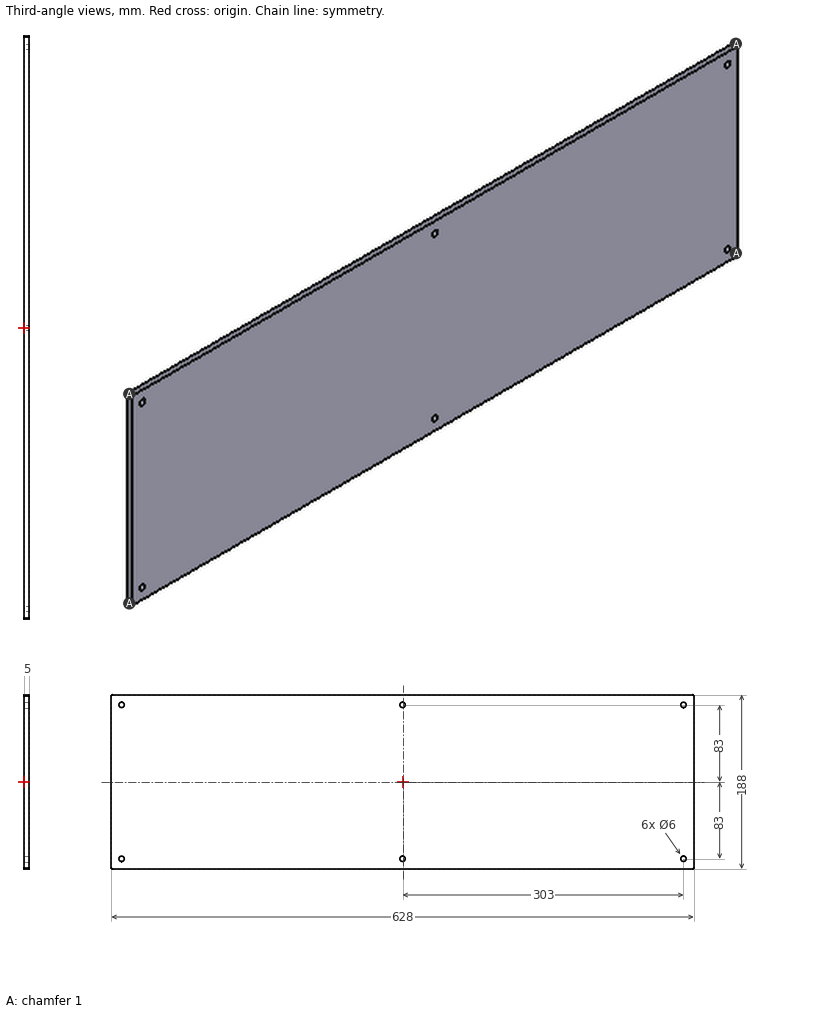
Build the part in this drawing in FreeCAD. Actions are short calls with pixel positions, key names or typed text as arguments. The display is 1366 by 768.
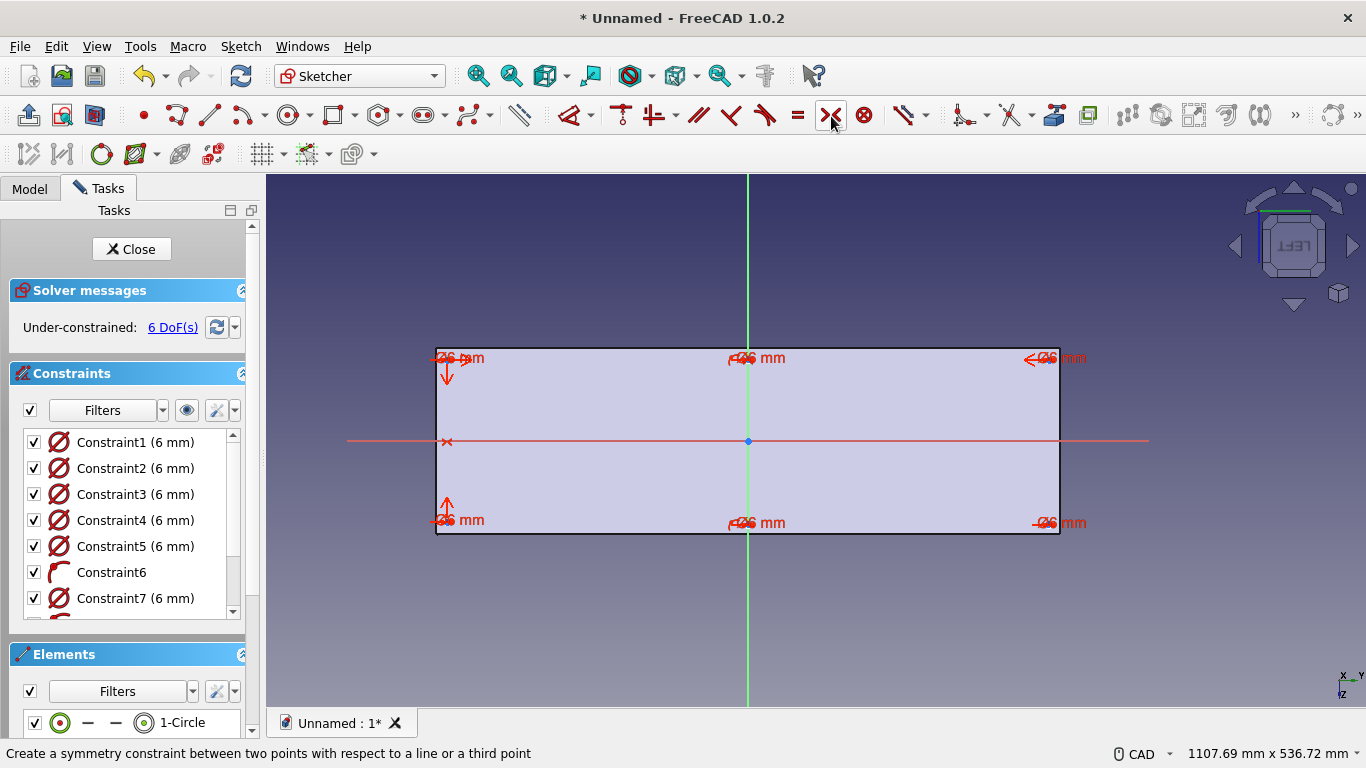
click(1049, 360)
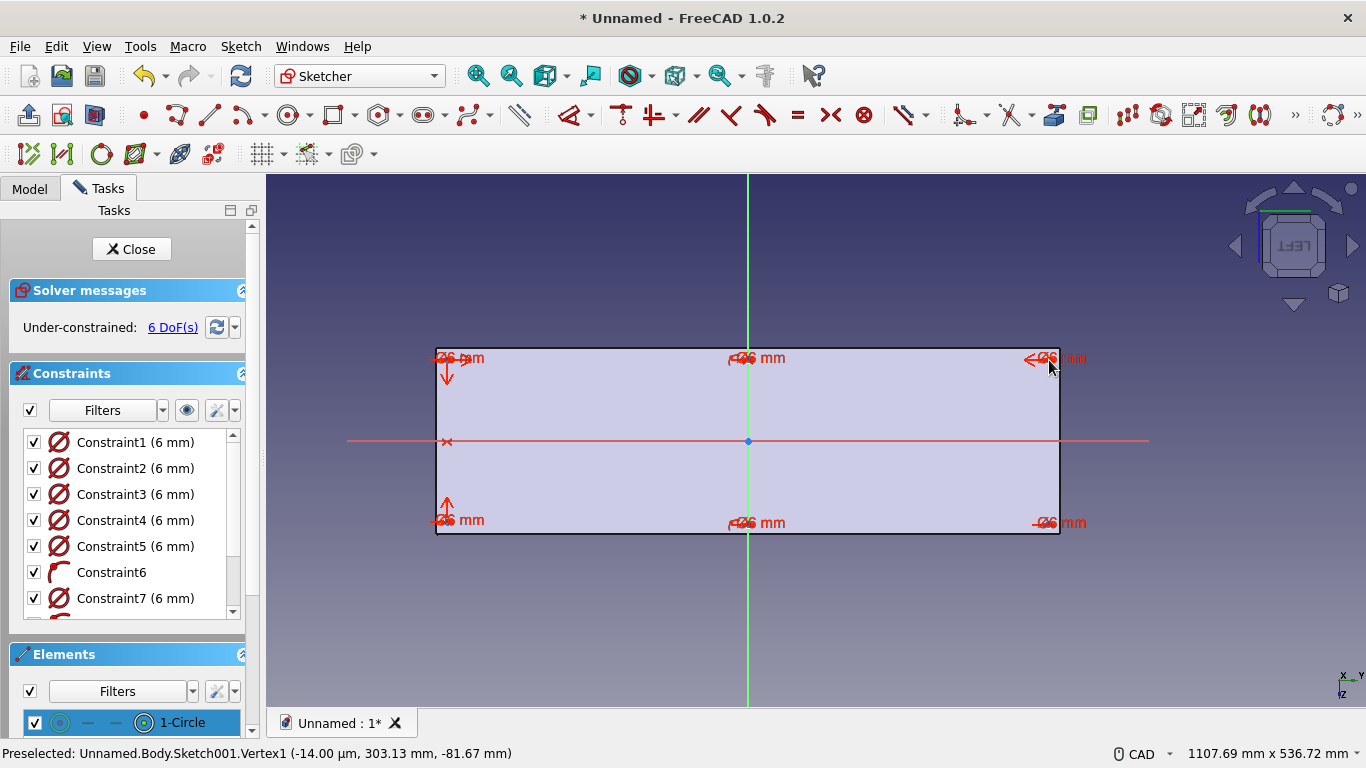
click(1049, 525)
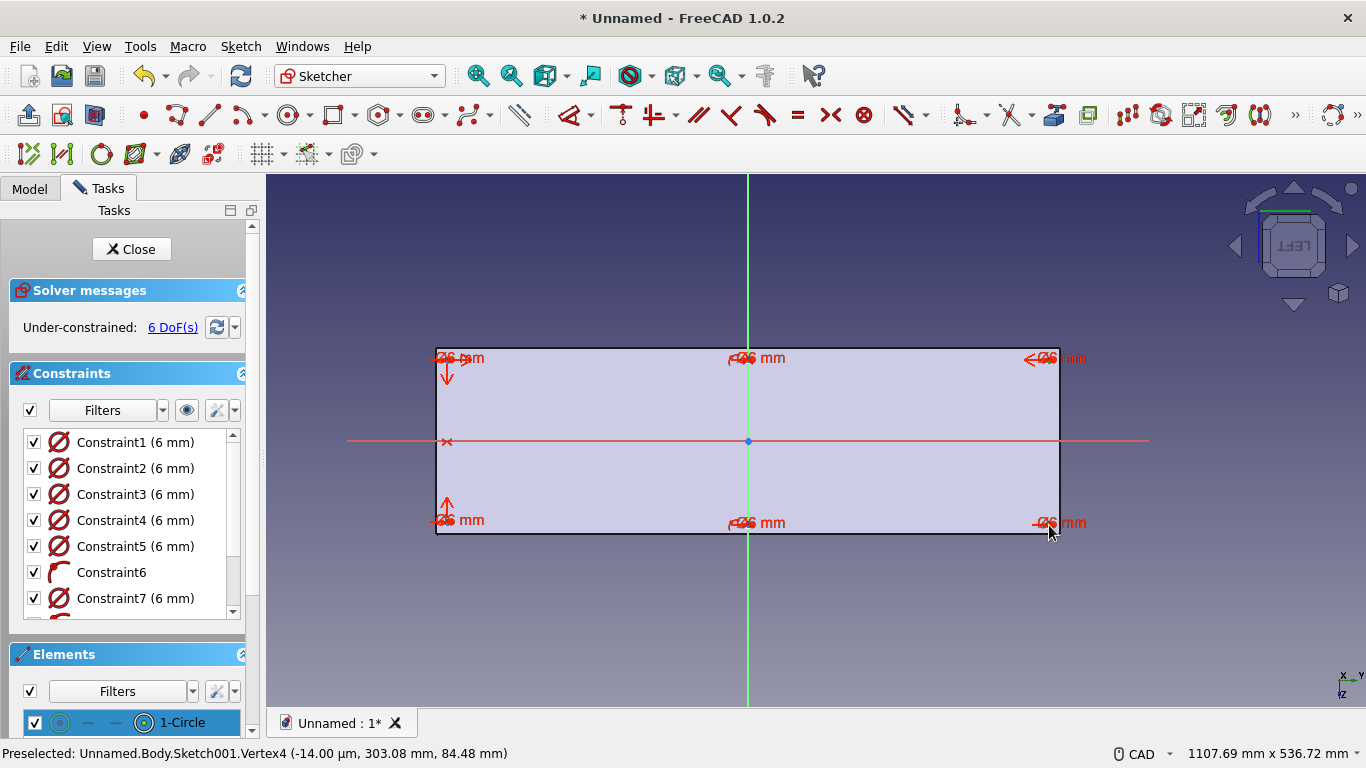
click(359, 441)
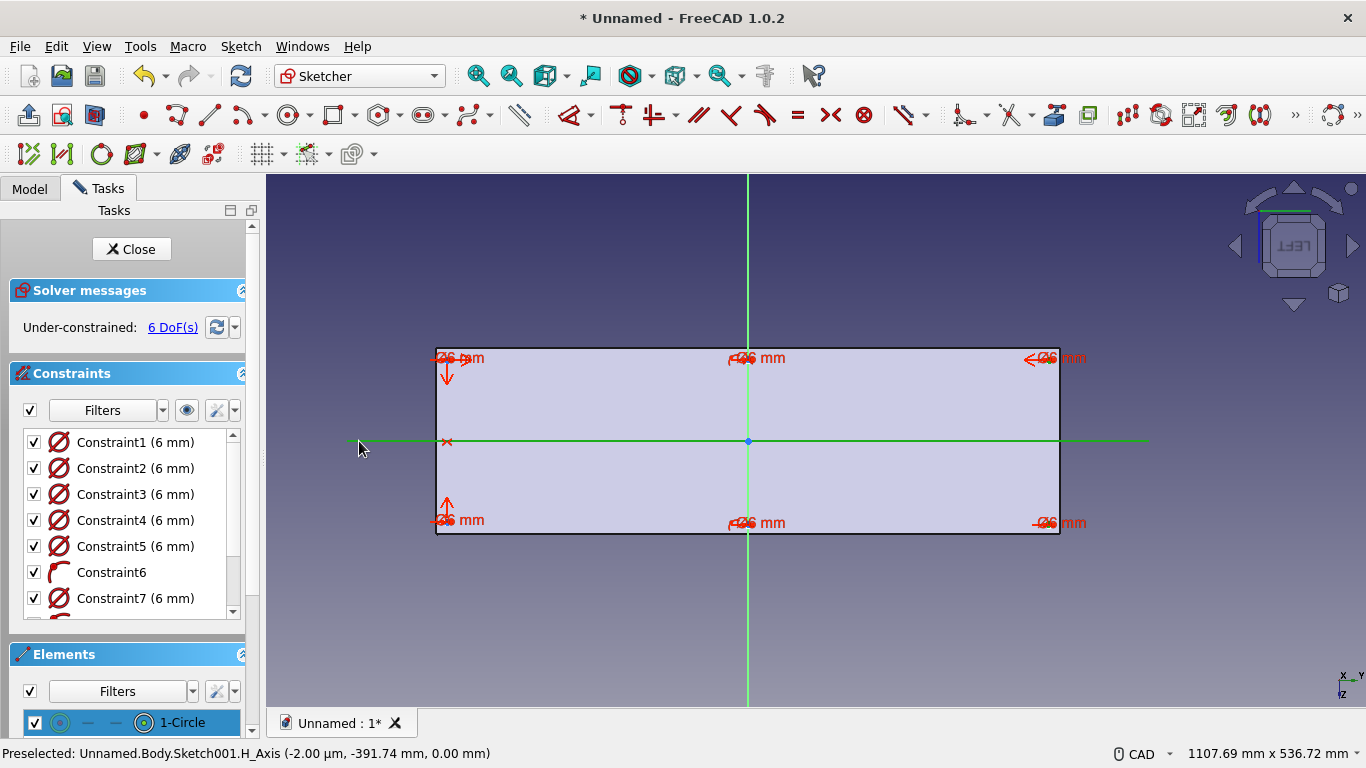
click(831, 116)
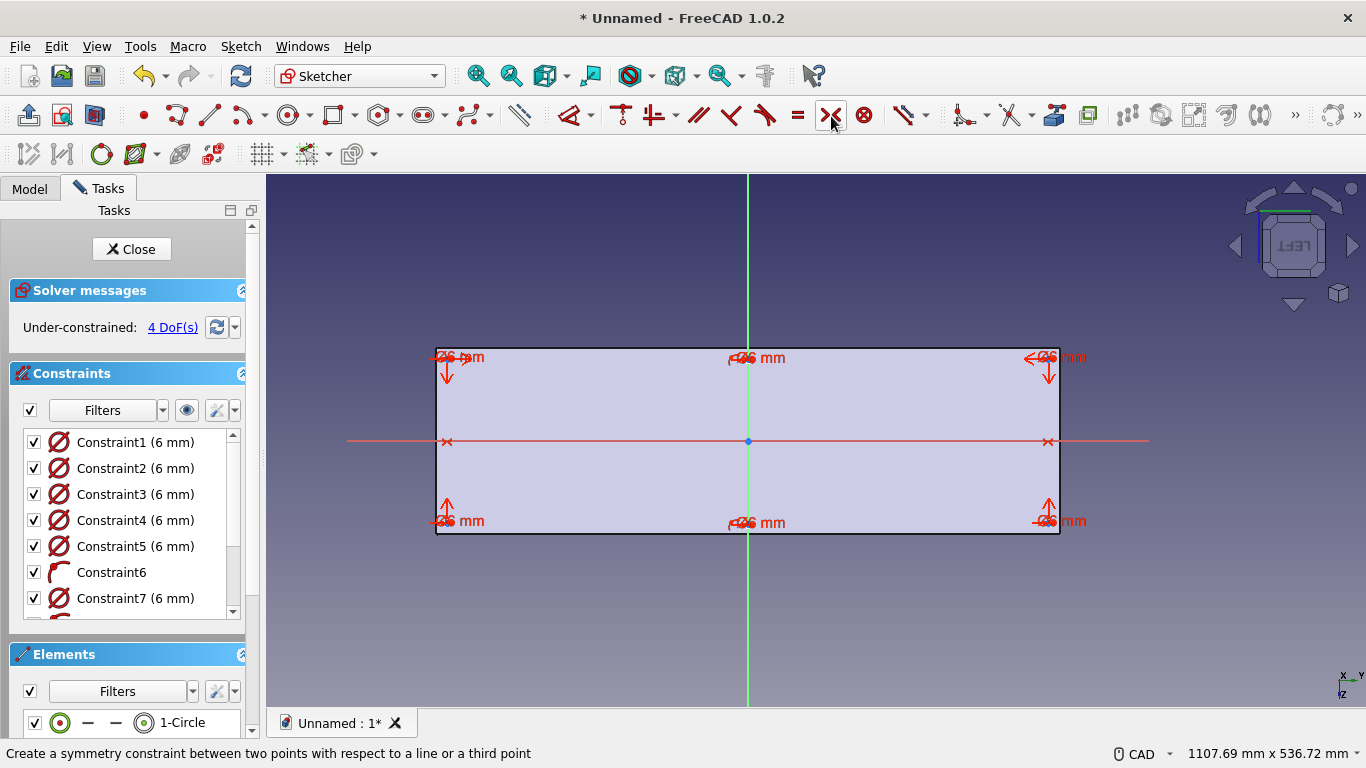
click(568, 116)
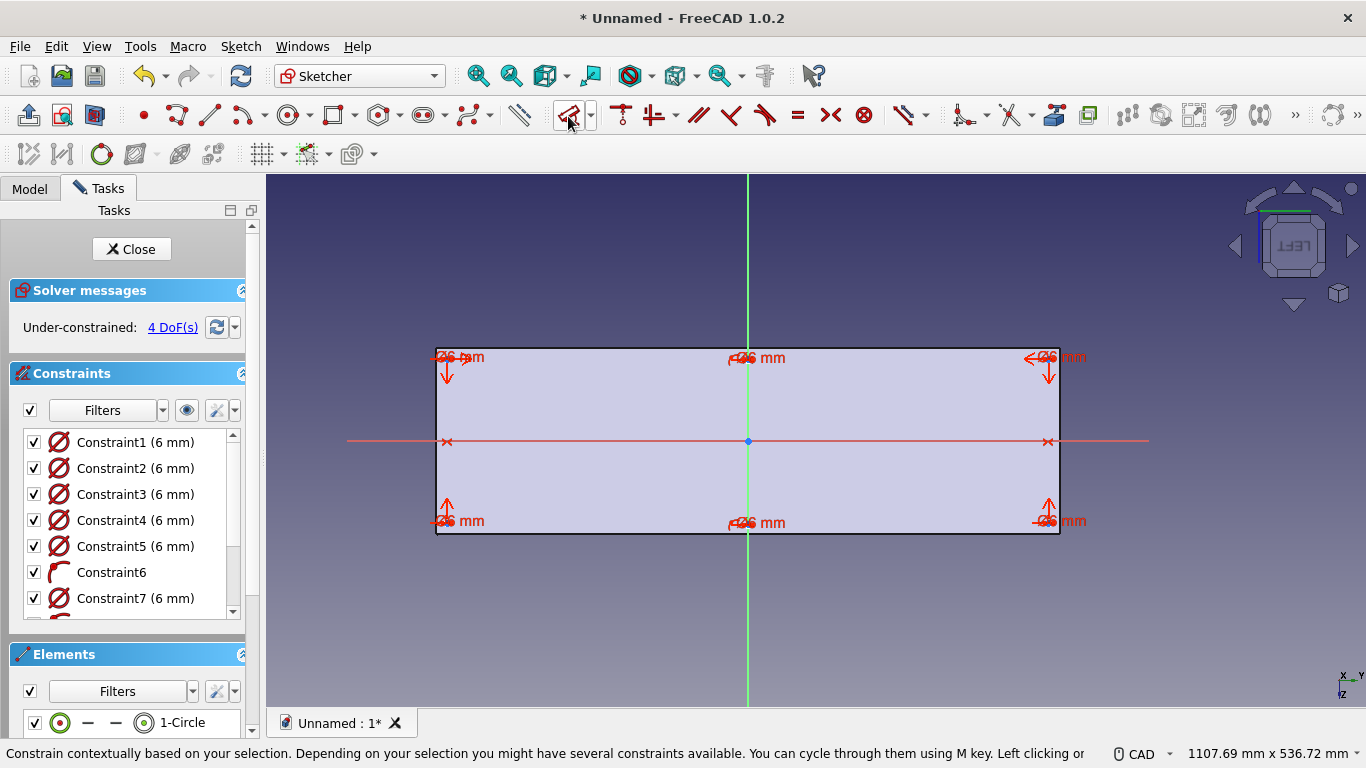
click(1049, 359)
click(1083, 400)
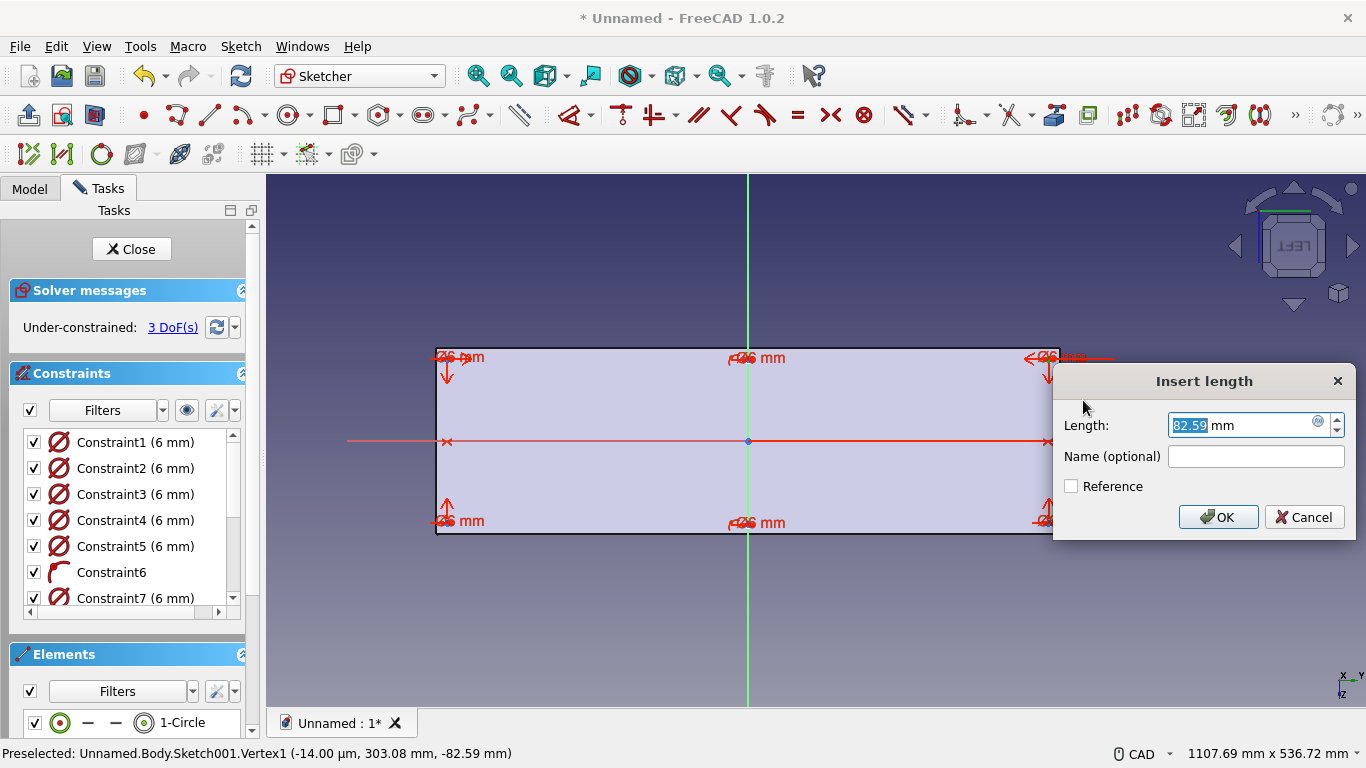
text(83)
key(Return)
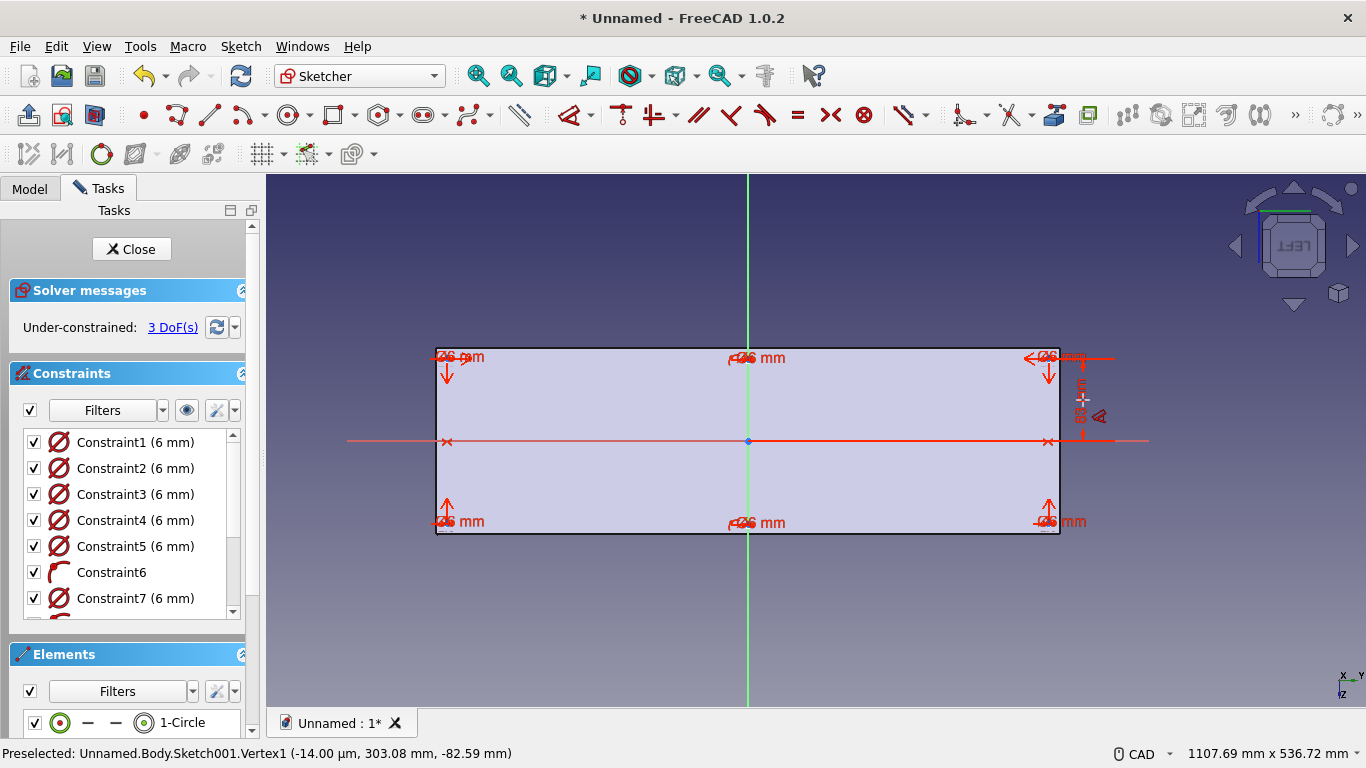
click(748, 525)
click(782, 483)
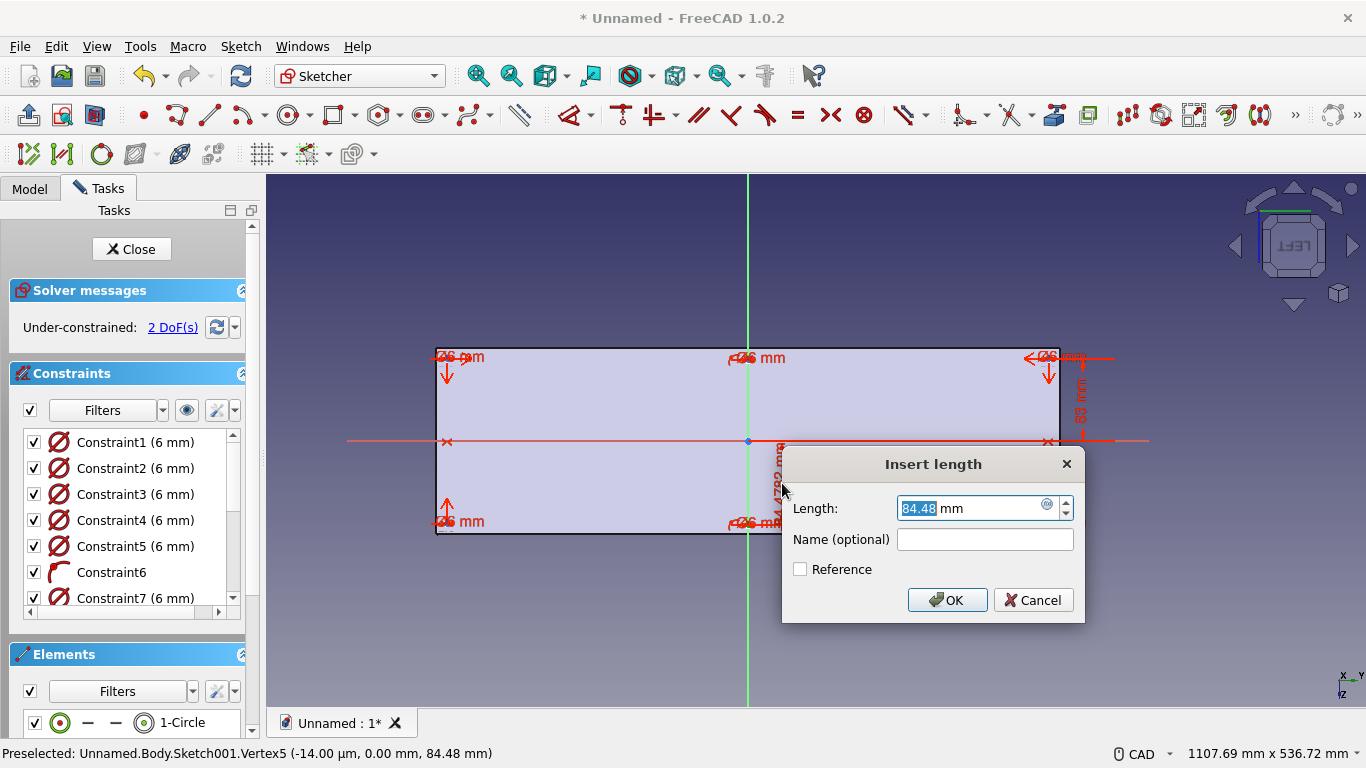
text(83)
key(Return)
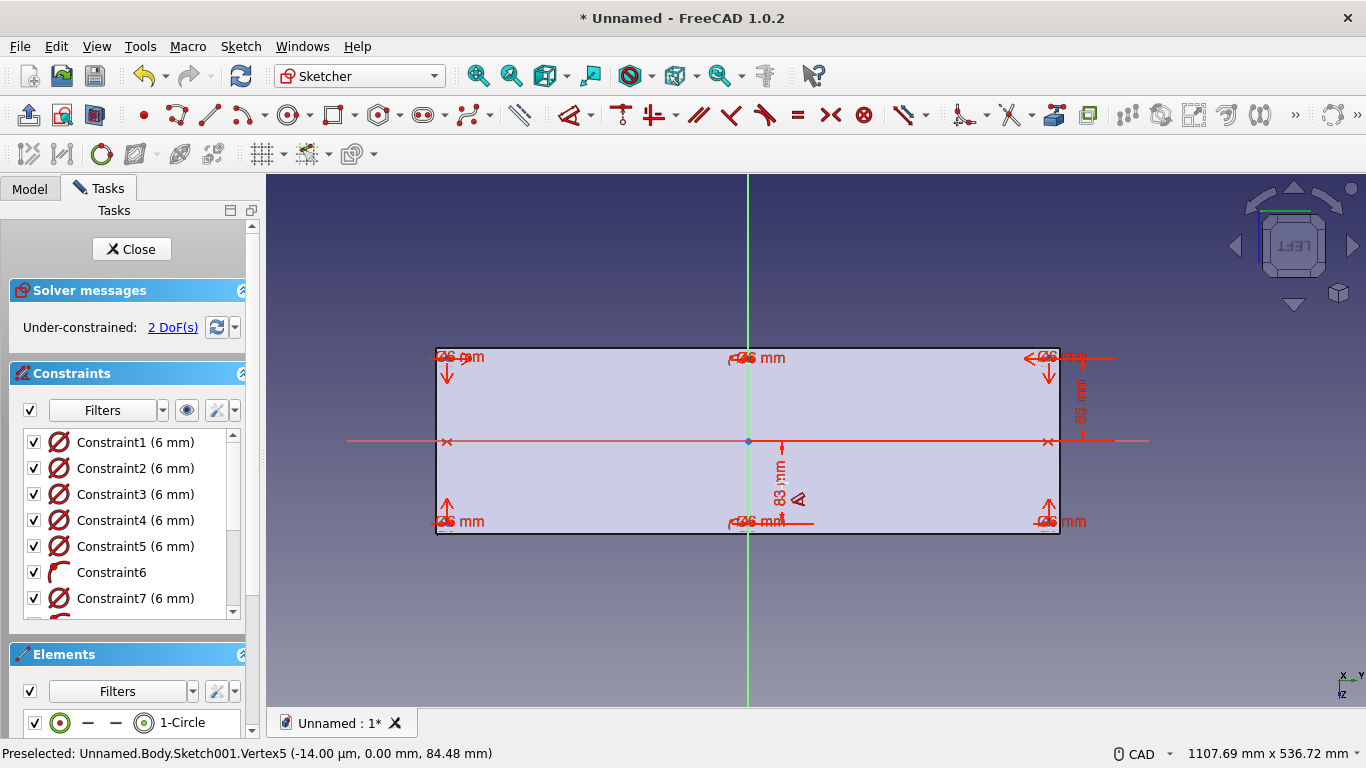
click(748, 360)
click(782, 401)